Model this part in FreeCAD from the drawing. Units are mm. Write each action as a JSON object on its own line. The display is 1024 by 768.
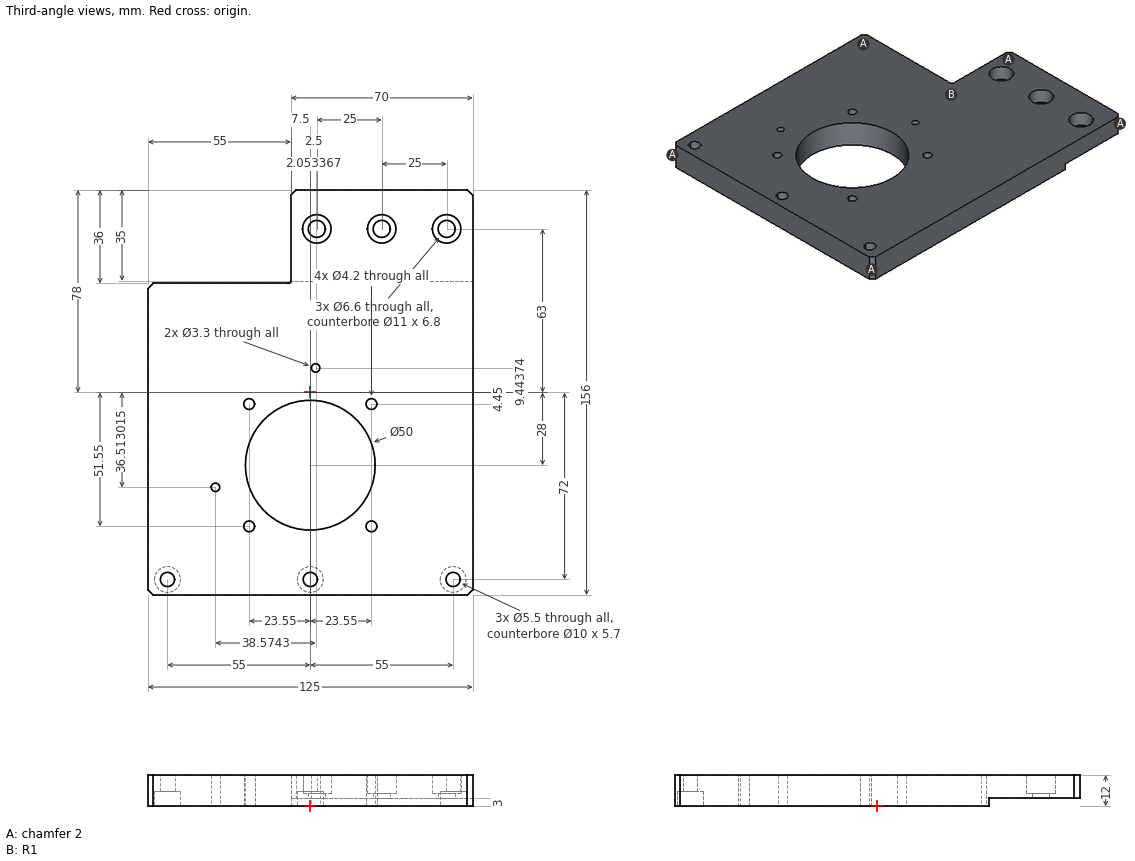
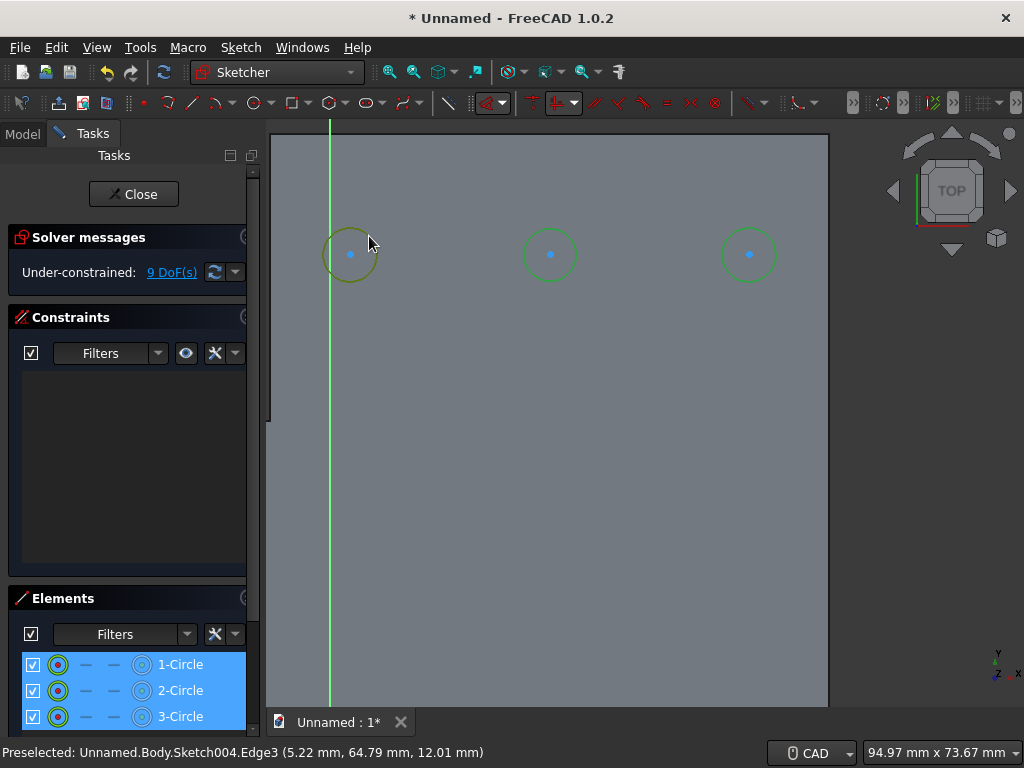
{"action": "left_click", "coordinate": [668, 104]}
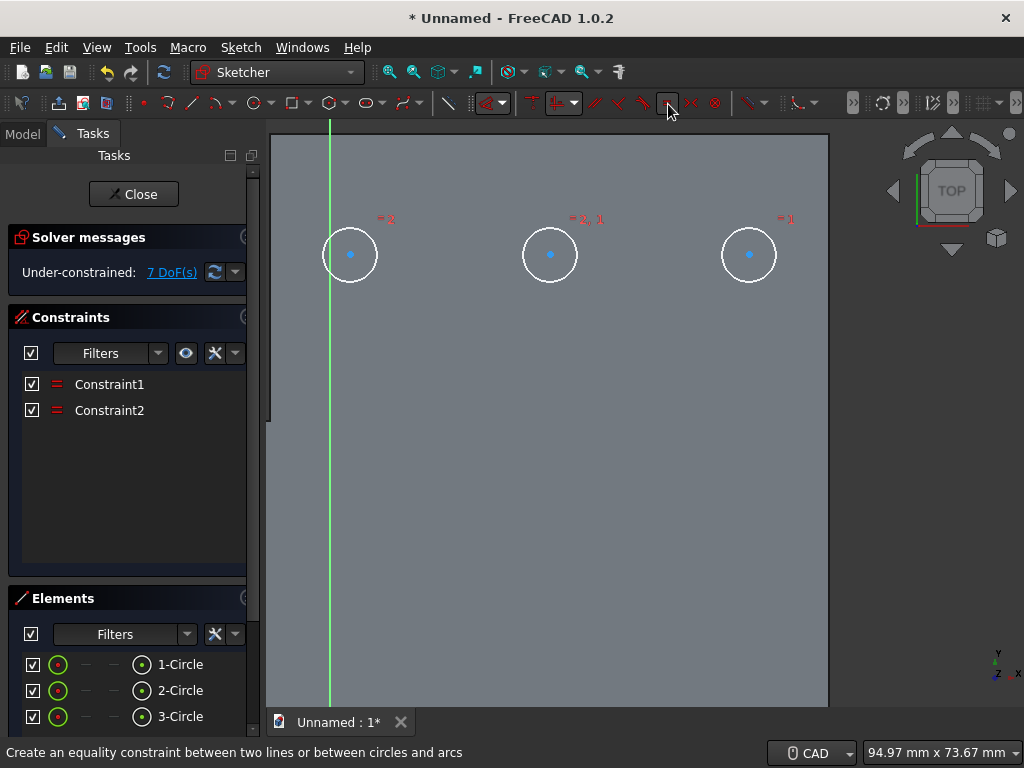
{"action": "left_click", "coordinate": [749, 255]}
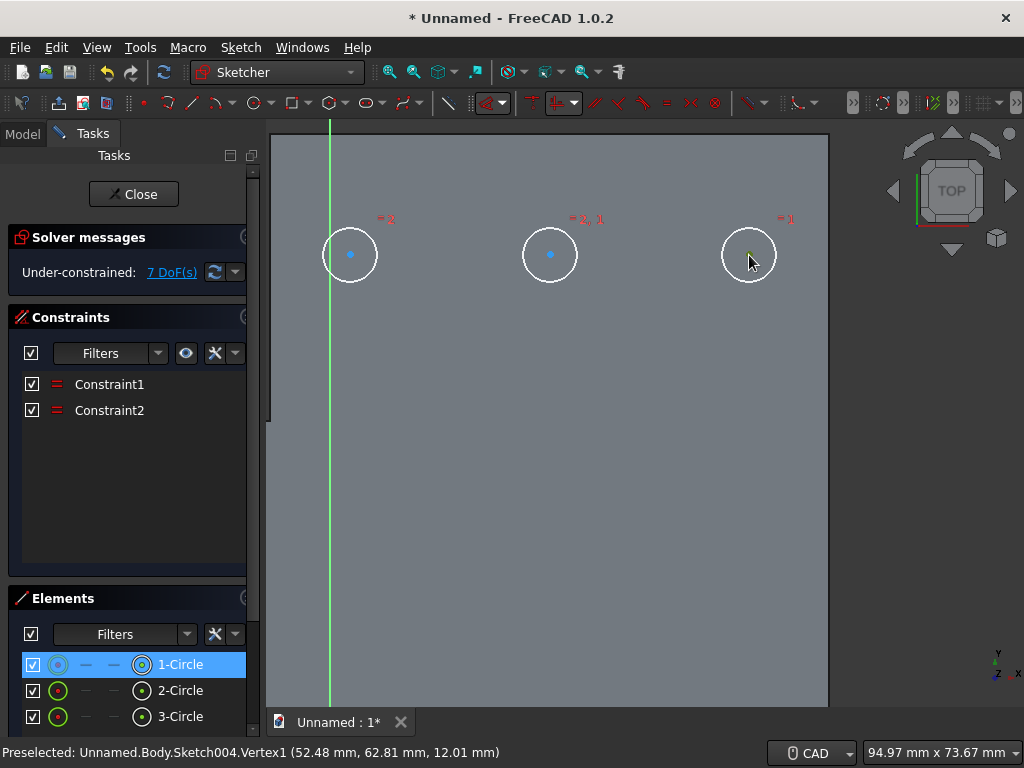
{"action": "left_click", "coordinate": [550, 255]}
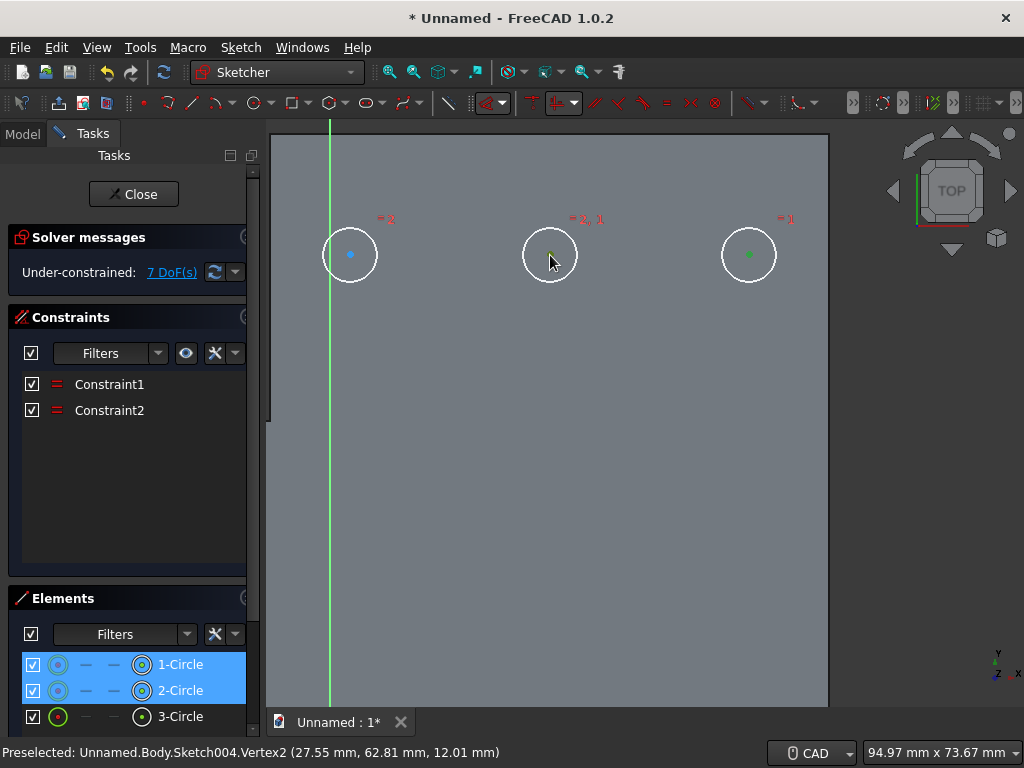
{"action": "left_click", "coordinate": [576, 104]}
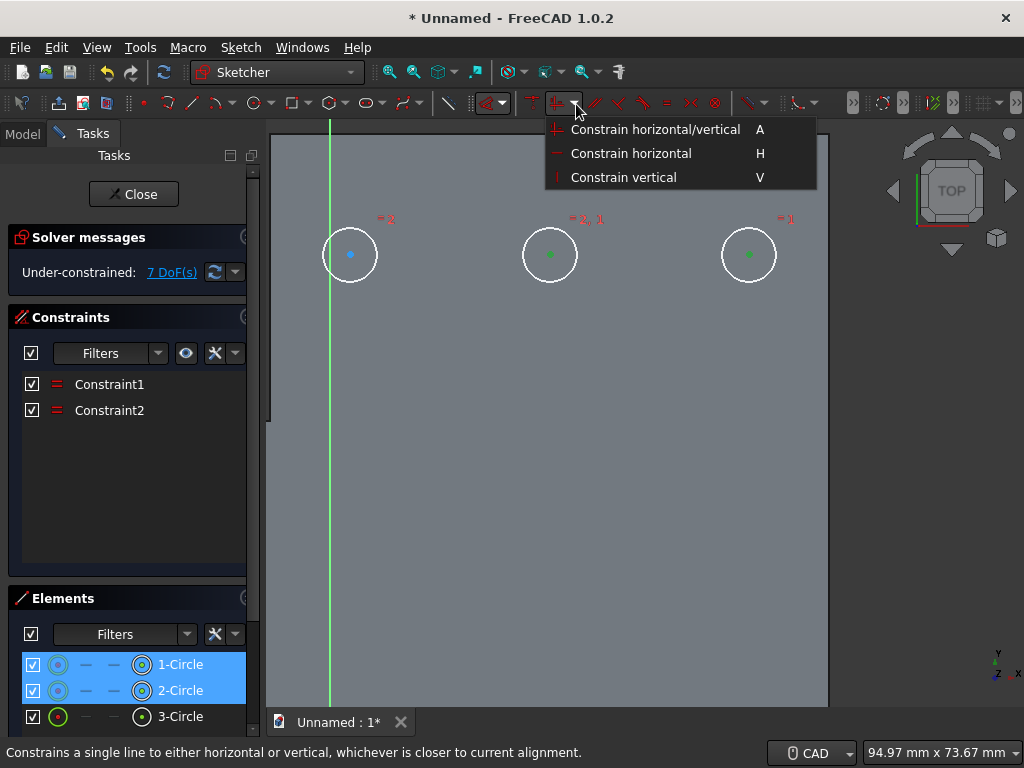
{"action": "left_click", "coordinate": [681, 153]}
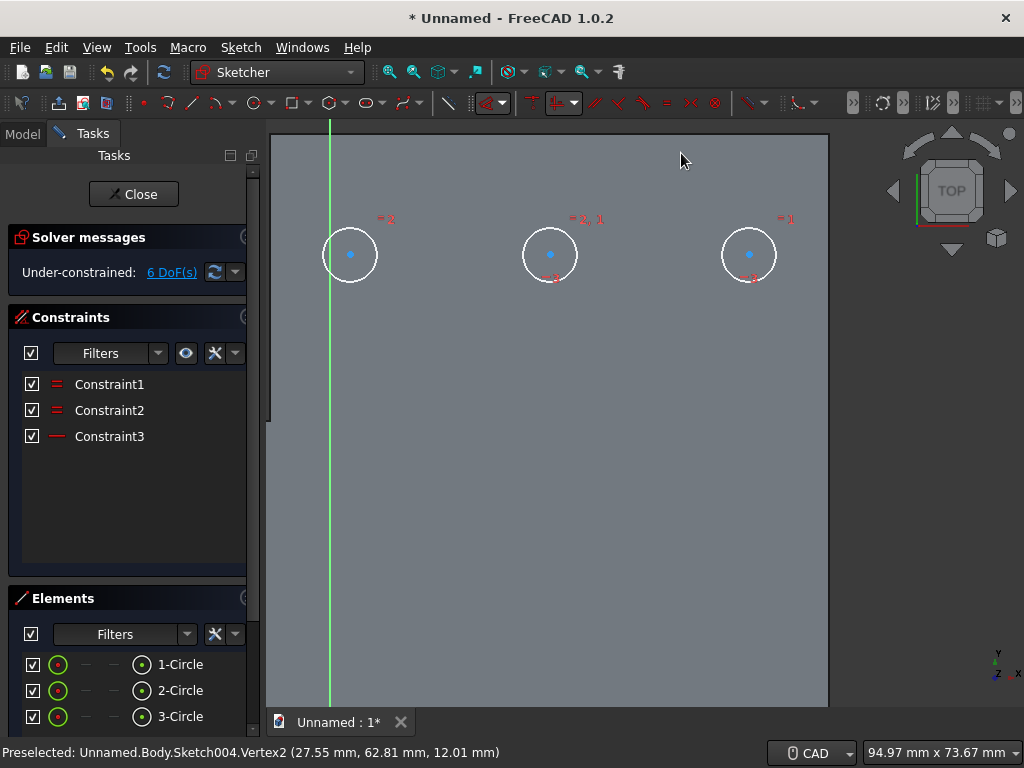
{"action": "left_click", "coordinate": [550, 255]}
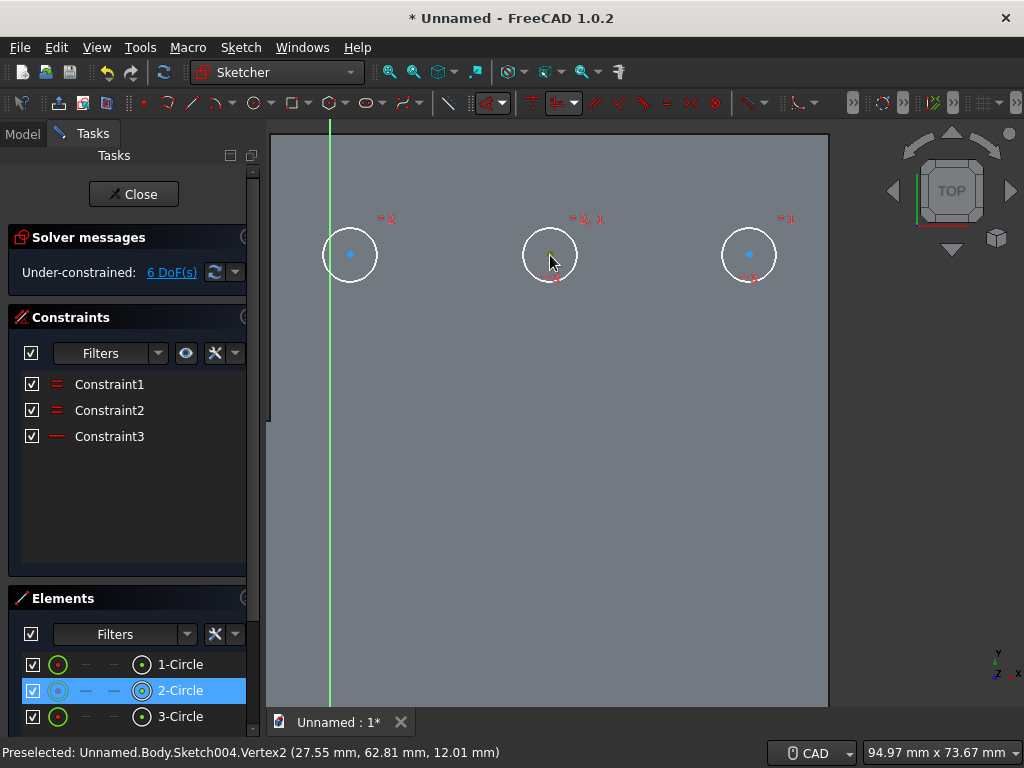
{"action": "left_click", "coordinate": [350, 255]}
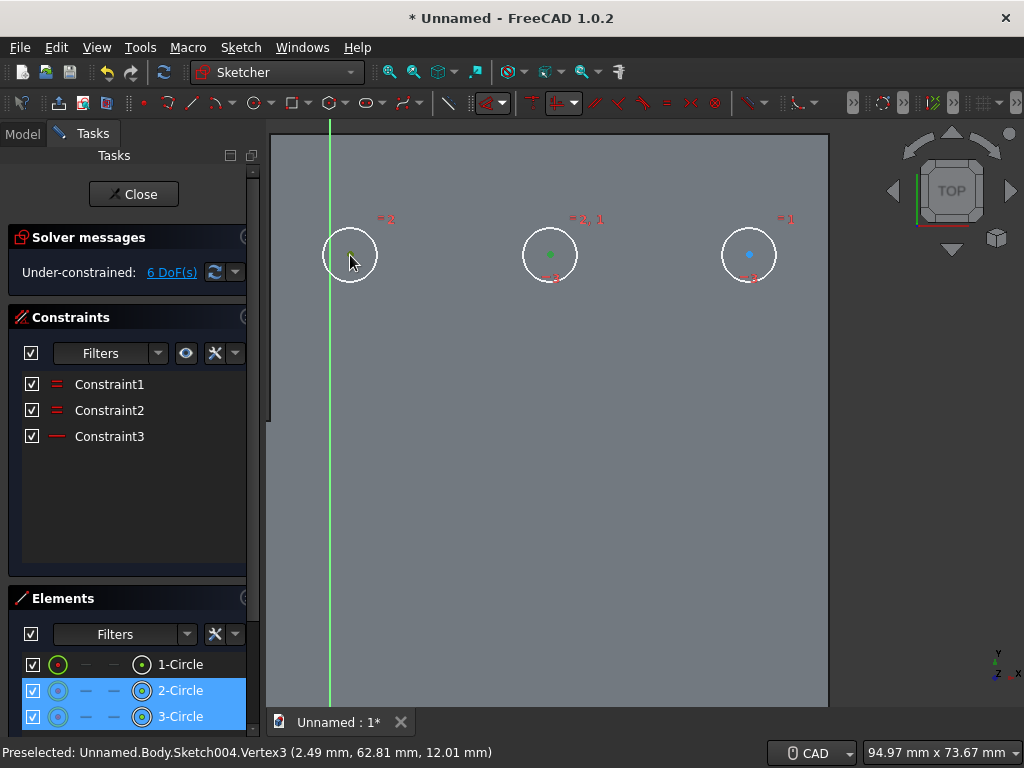
{"action": "left_click", "coordinate": [576, 104]}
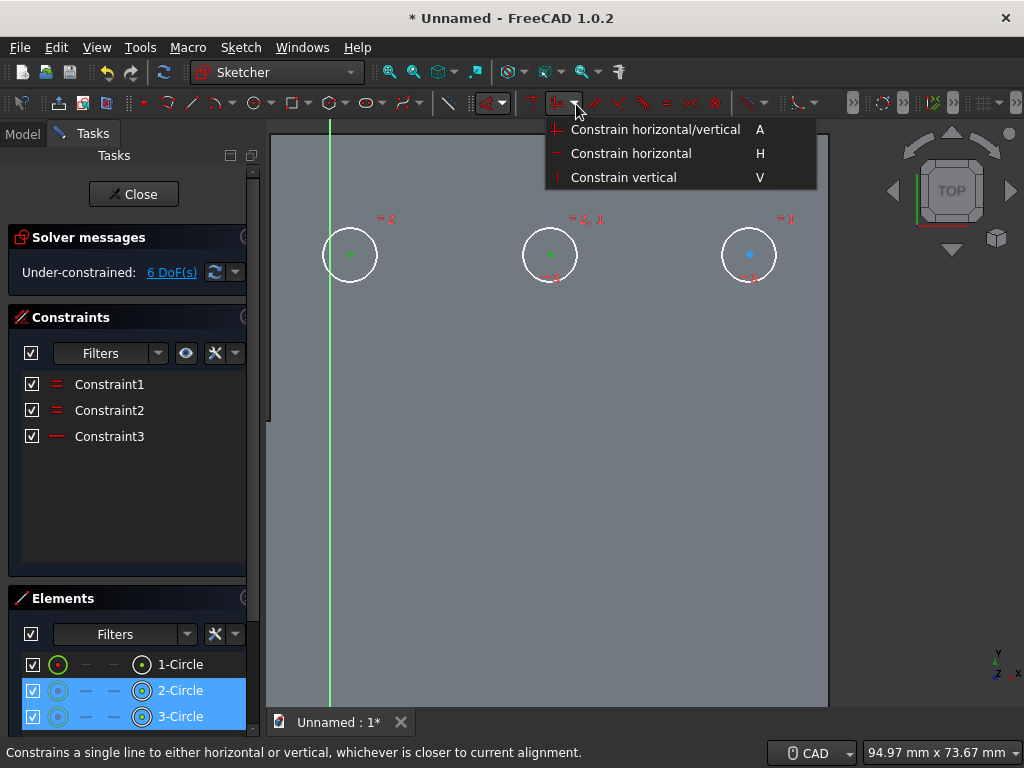
{"action": "left_click", "coordinate": [681, 153]}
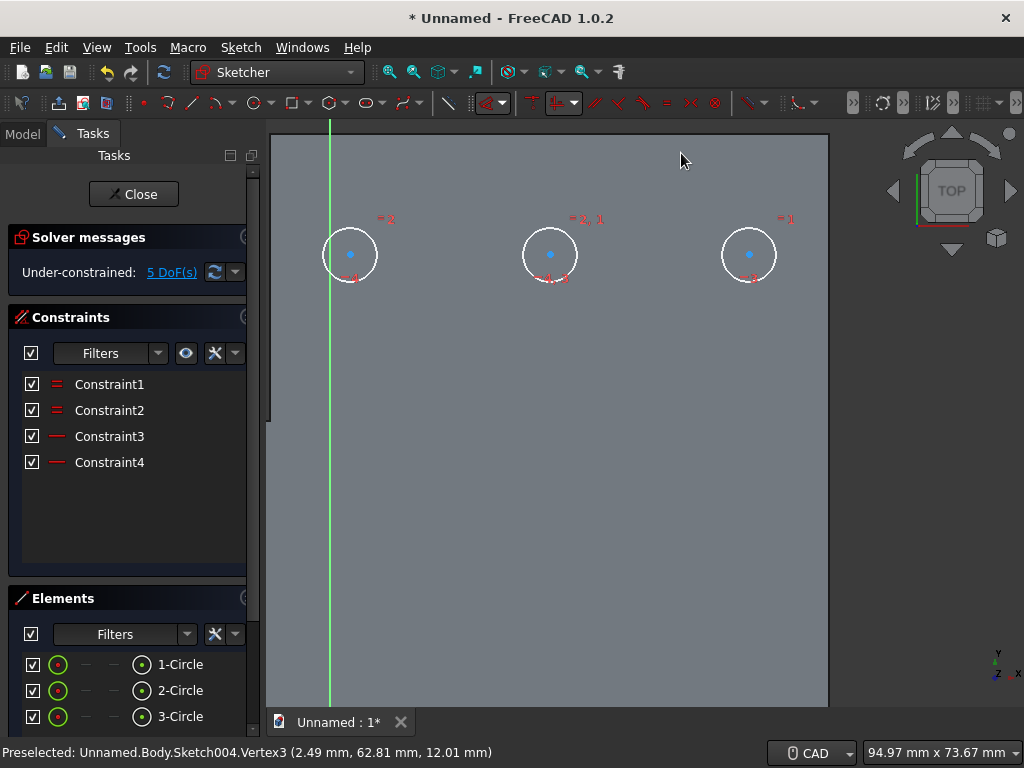
{"action": "left_click", "coordinate": [768, 236]}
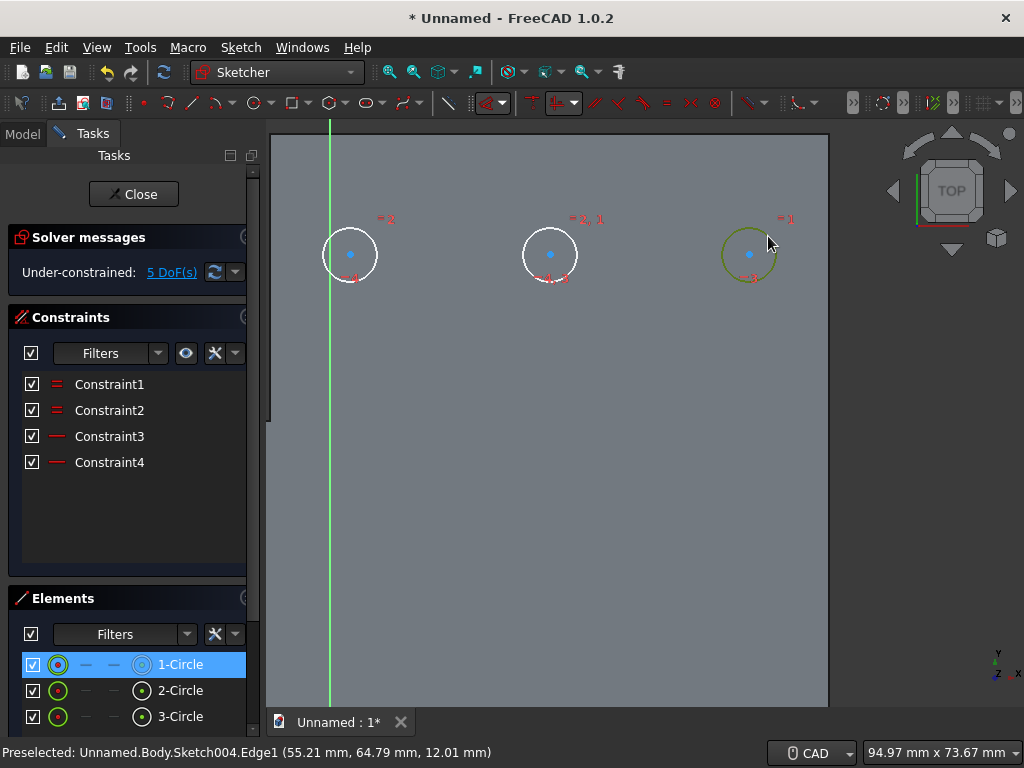
{"action": "left_click", "coordinate": [504, 104]}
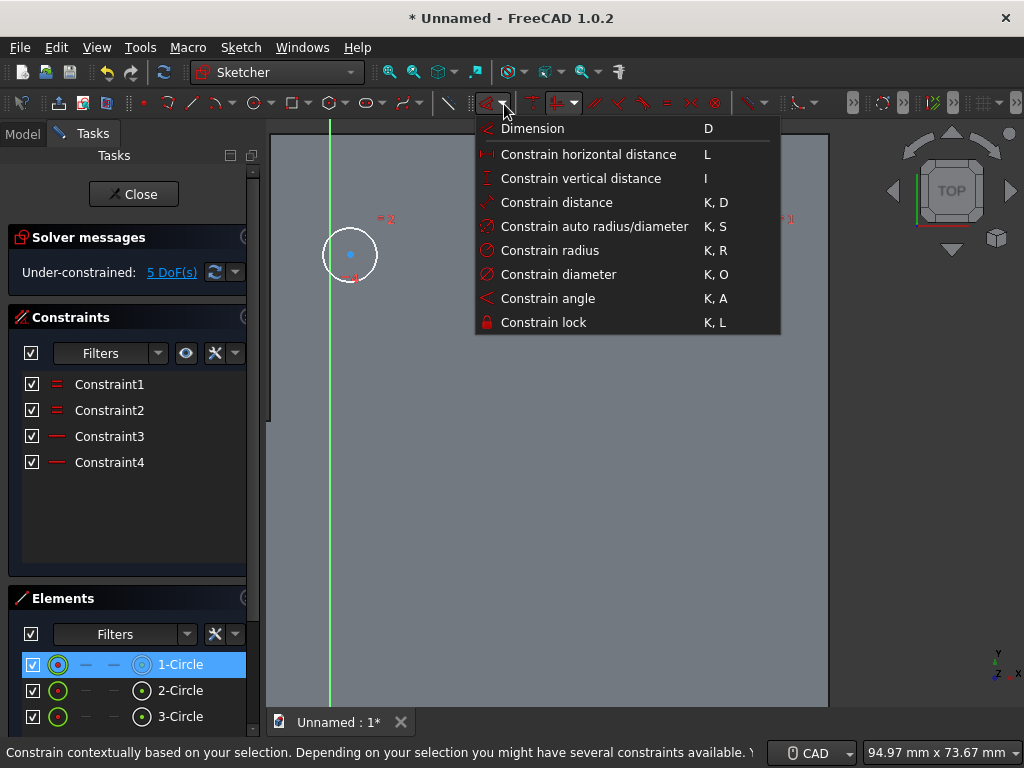
{"action": "left_click", "coordinate": [628, 274]}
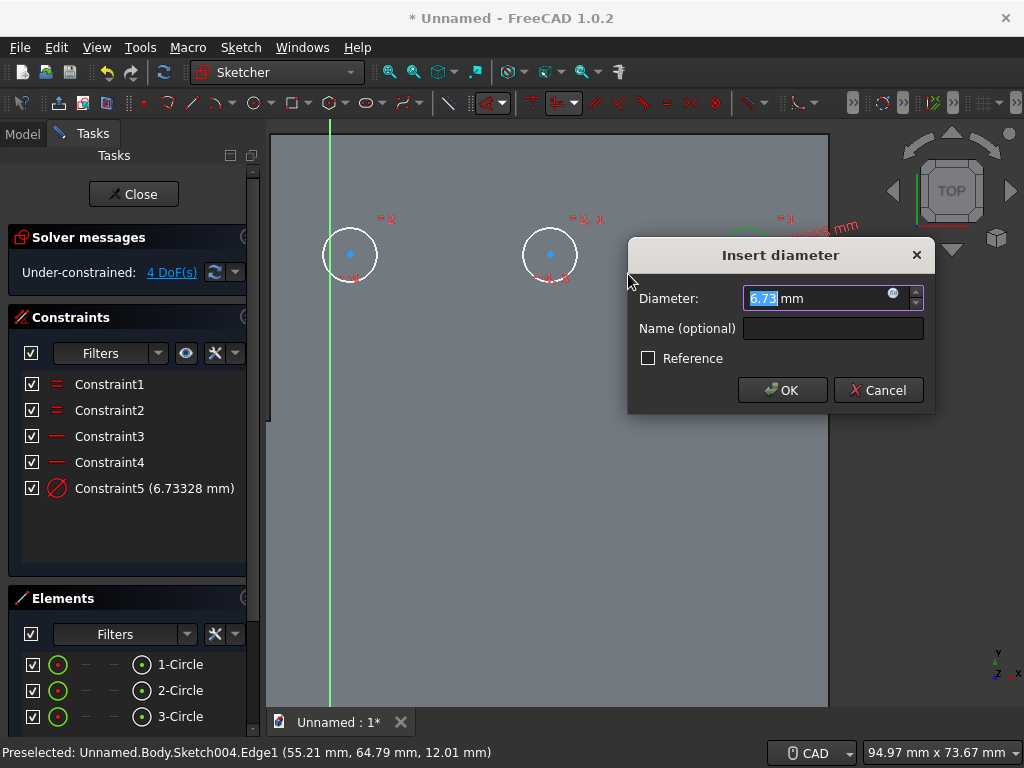
{"action": "type", "text": "6.6"}
{"action": "key", "text": "Return"}